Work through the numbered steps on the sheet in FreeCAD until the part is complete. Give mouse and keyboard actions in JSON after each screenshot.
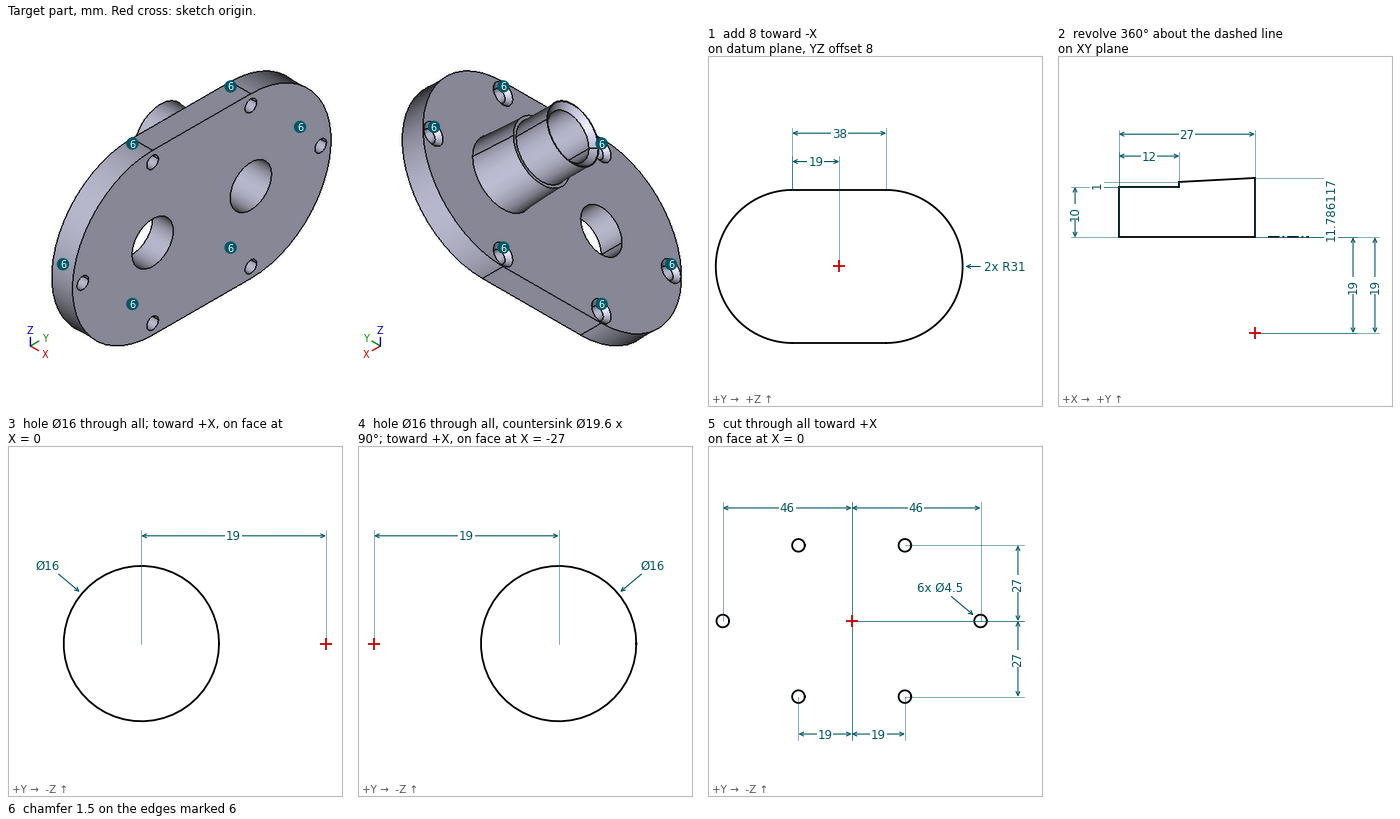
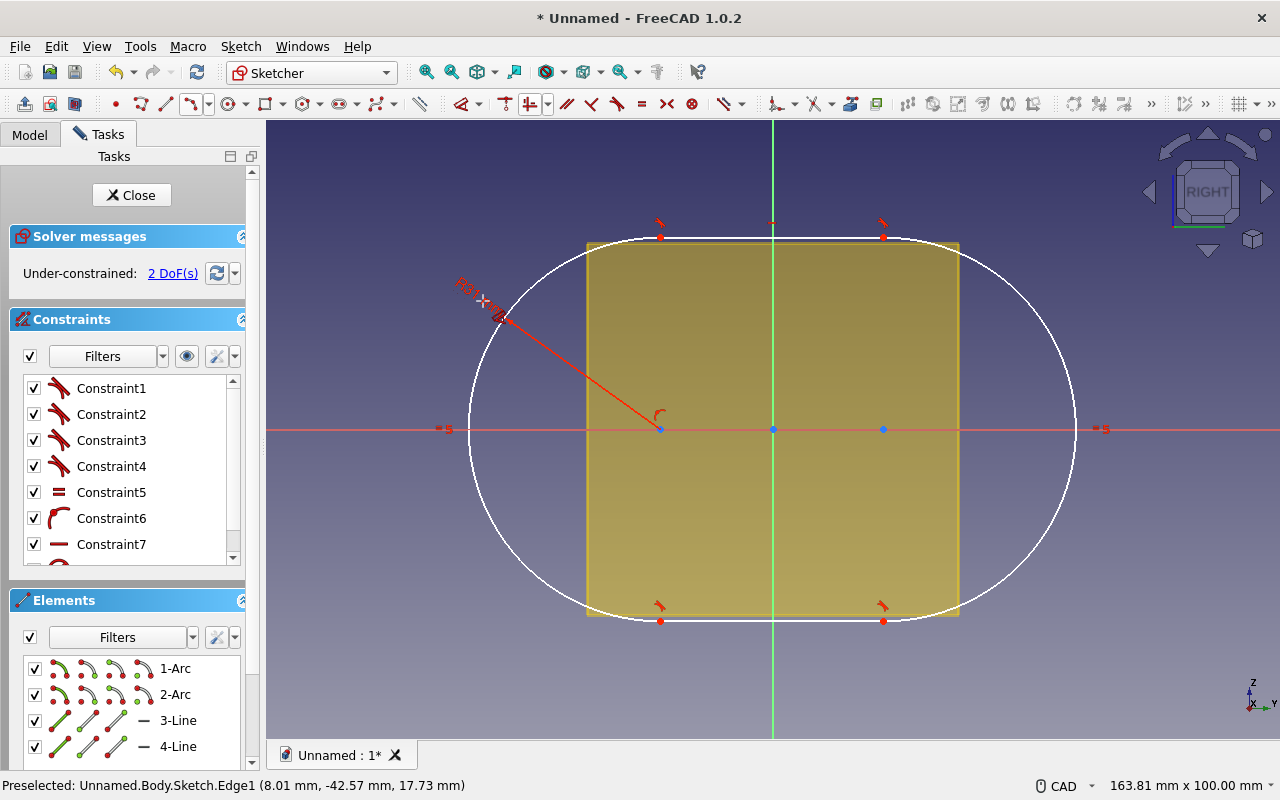
{"action": "left_click", "coordinate": [728, 238]}
{"action": "left_click", "coordinate": [721, 204]}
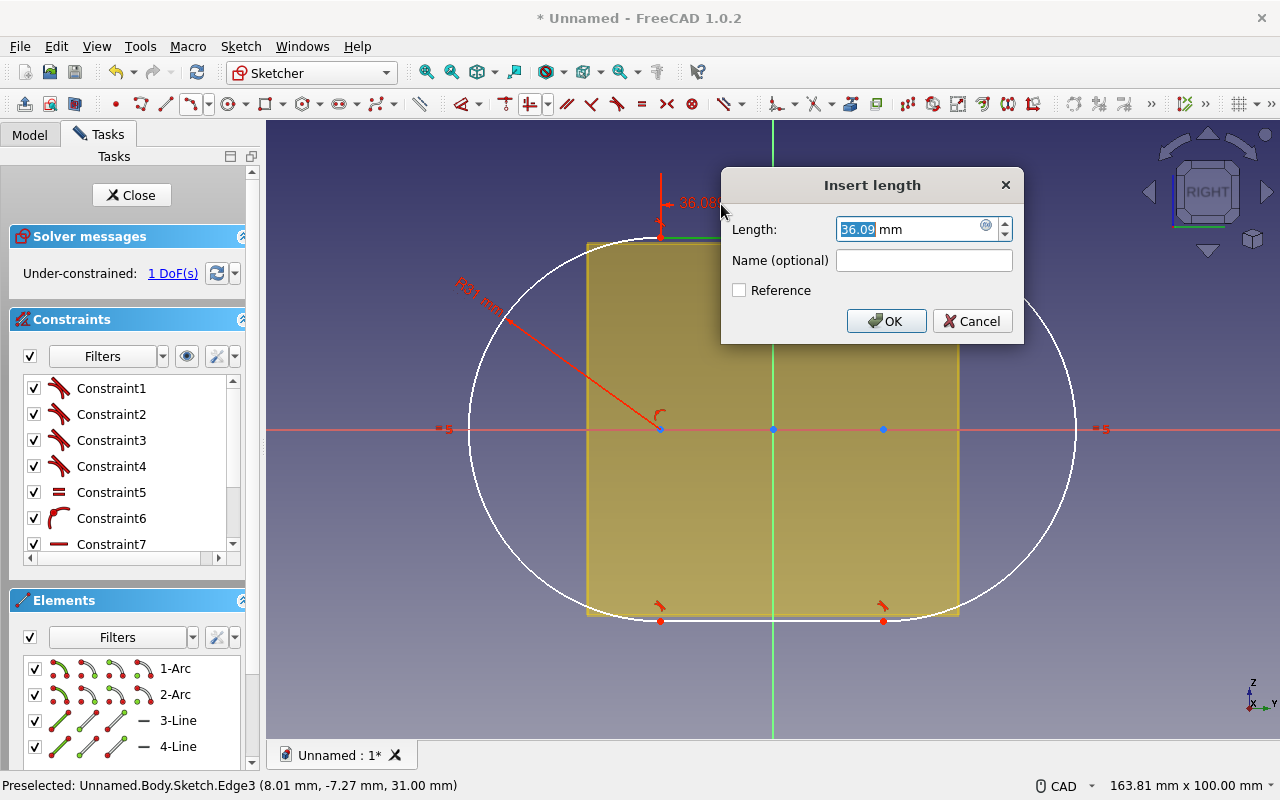
{"action": "type", "text": "38"}
{"action": "key", "text": "Return"}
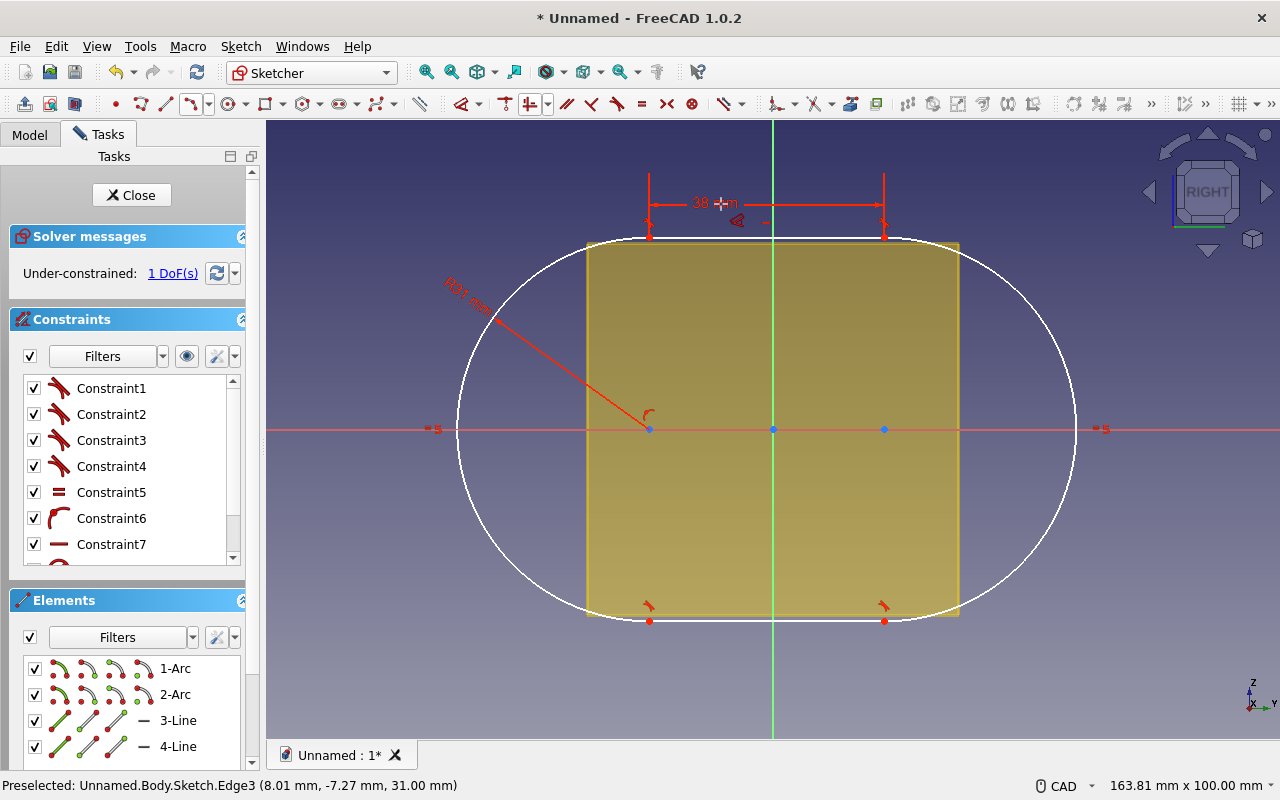
{"action": "left_click", "coordinate": [649, 238]}
{"action": "left_click", "coordinate": [711, 464]}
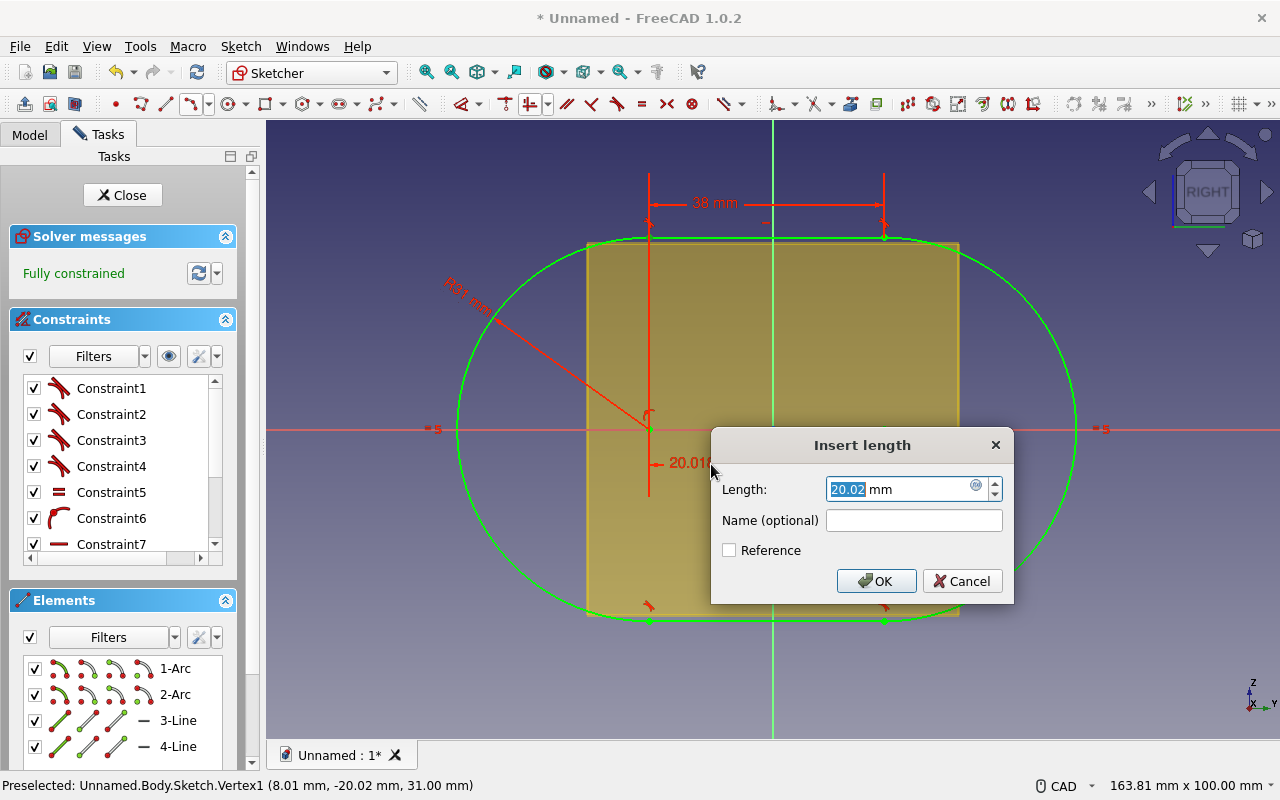
{"action": "type", "text": "19"}
{"action": "key", "text": "Return"}
{"action": "key", "text": "Escape"}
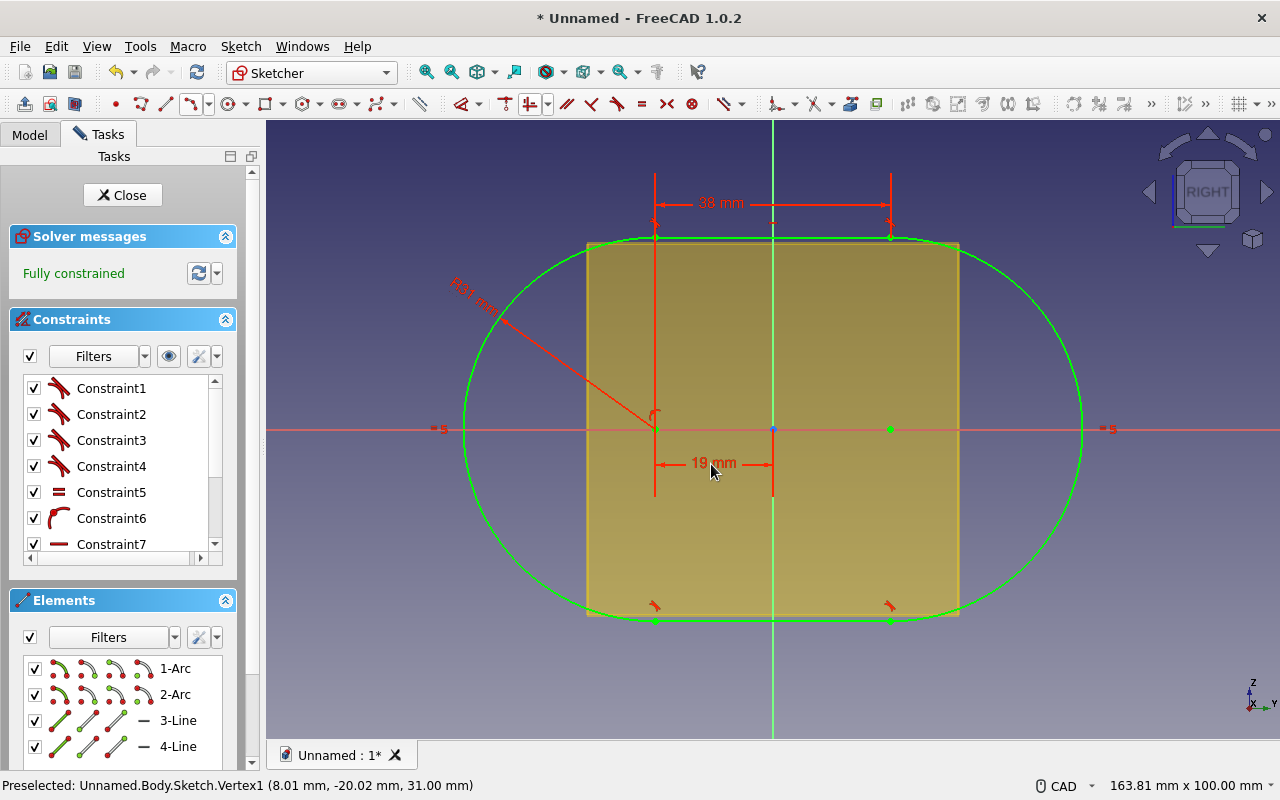
{"action": "left_click", "coordinate": [123, 195]}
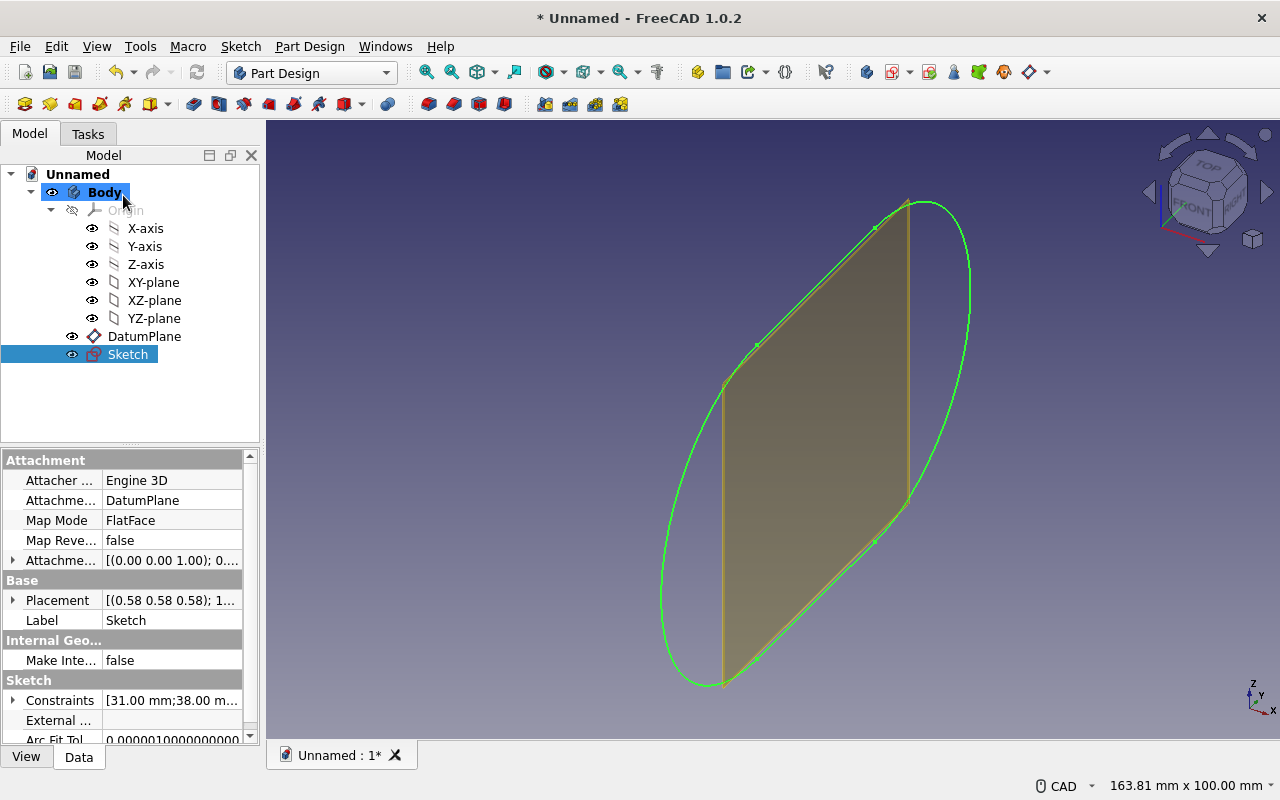
{"action": "left_click", "coordinate": [25, 104]}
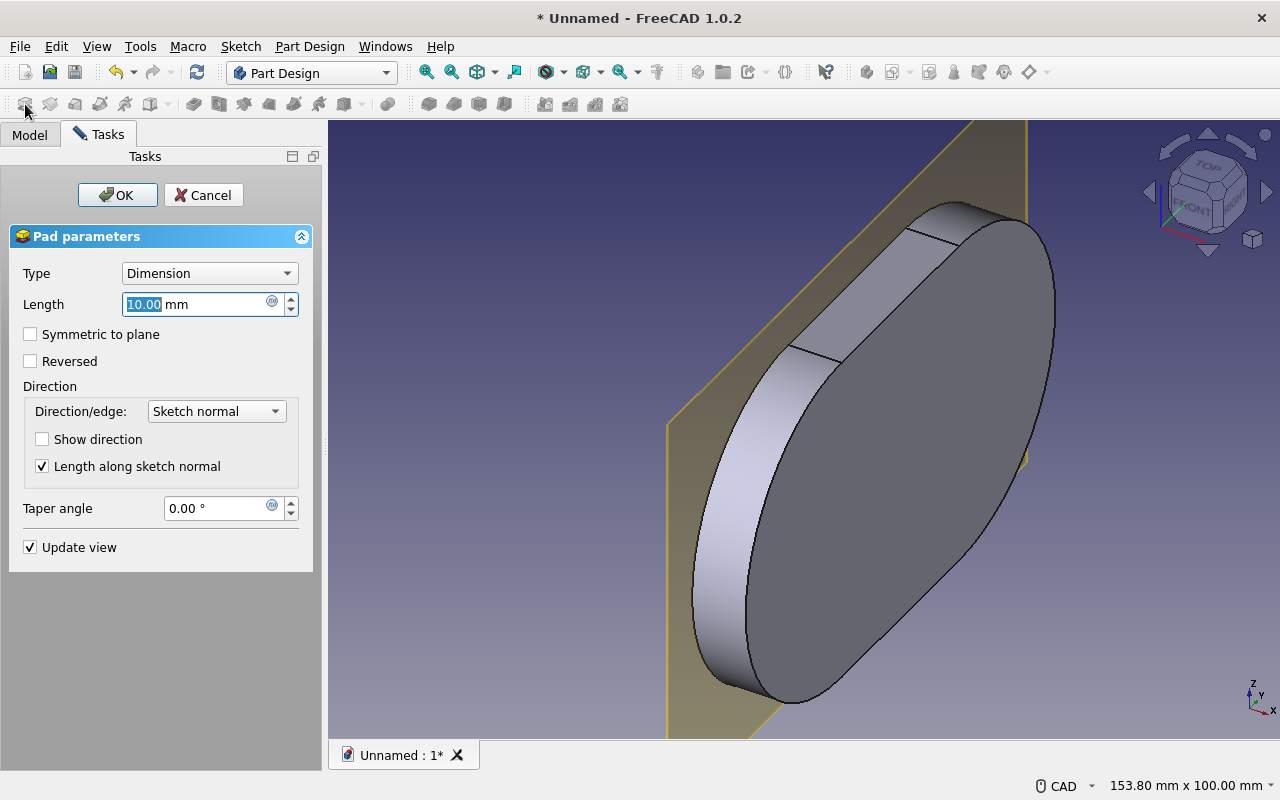
{"action": "type", "text": "8"}
{"action": "key", "text": "Tab"}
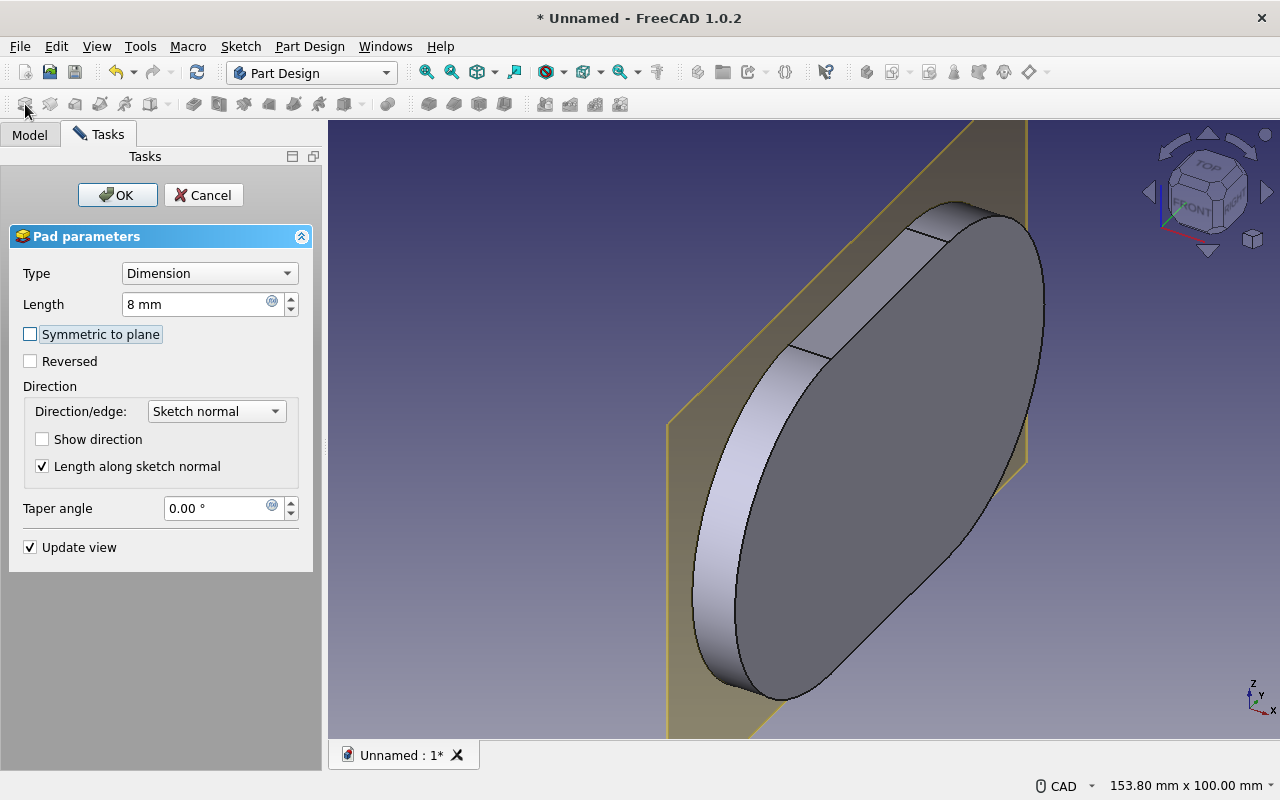
{"action": "left_click", "coordinate": [31, 361]}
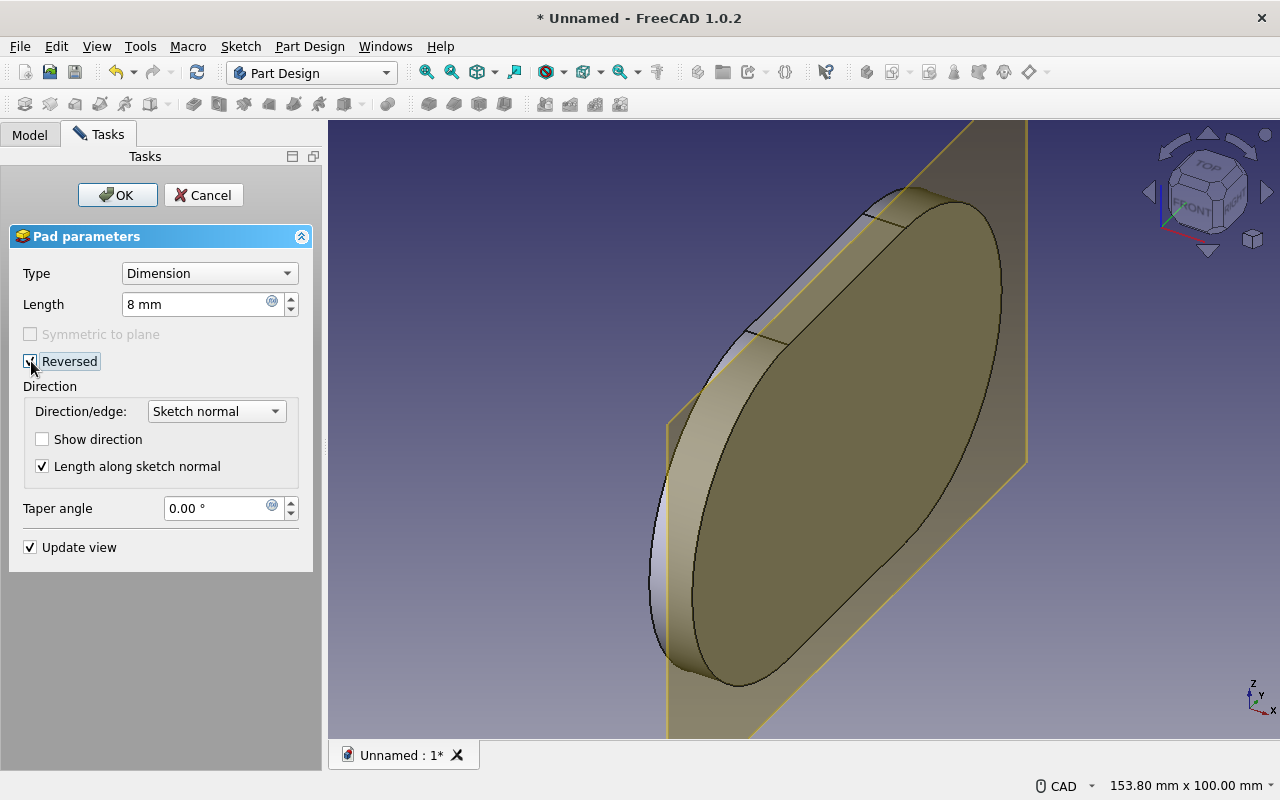
{"action": "left_click", "coordinate": [118, 195]}